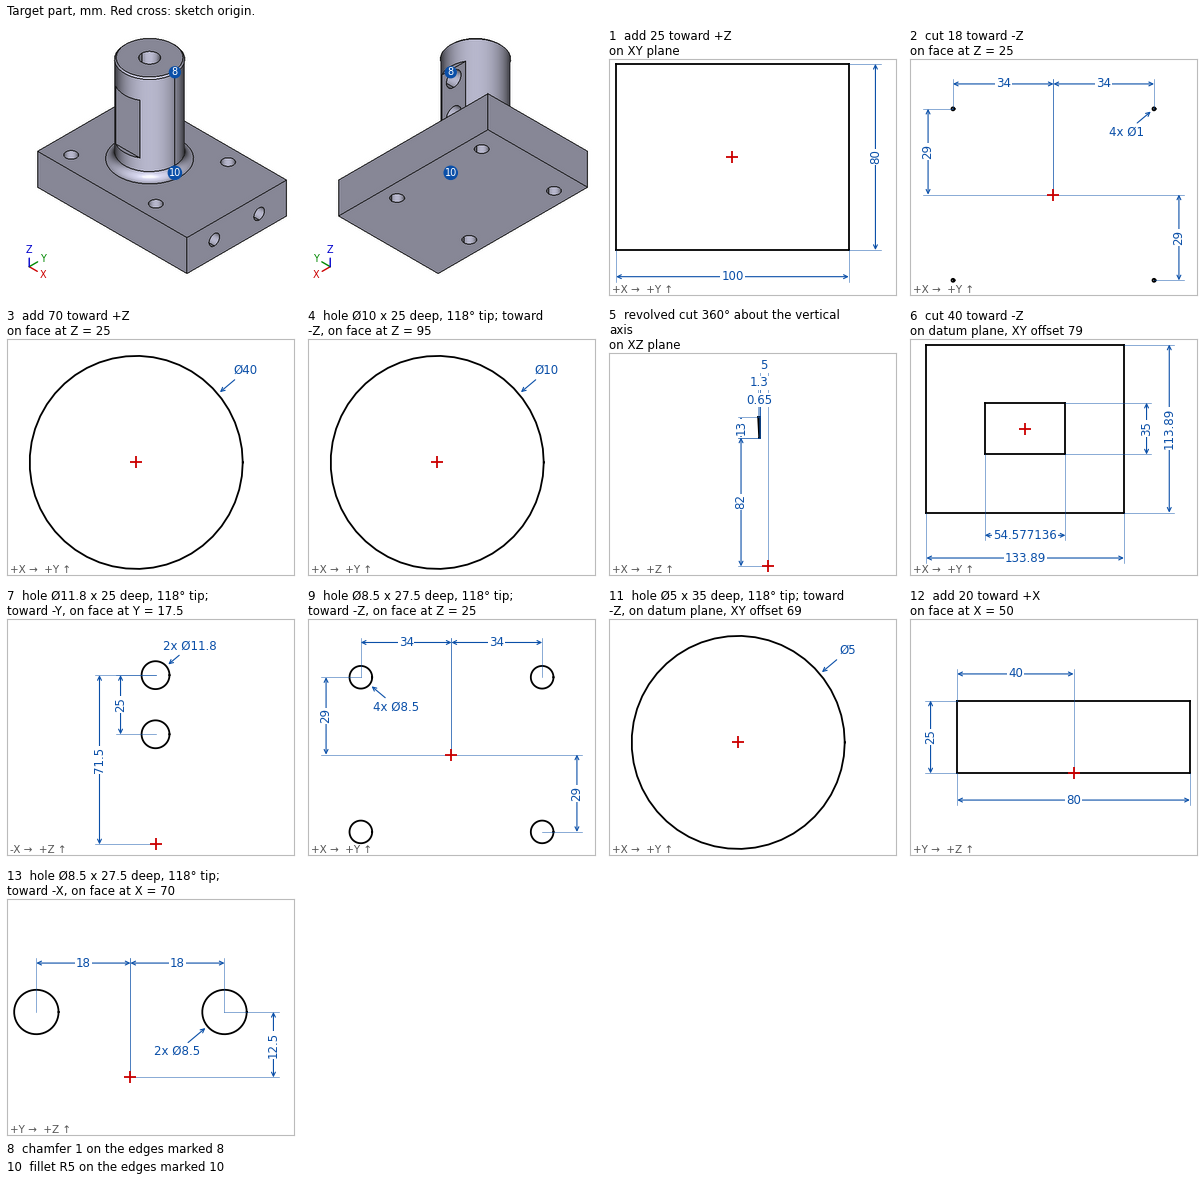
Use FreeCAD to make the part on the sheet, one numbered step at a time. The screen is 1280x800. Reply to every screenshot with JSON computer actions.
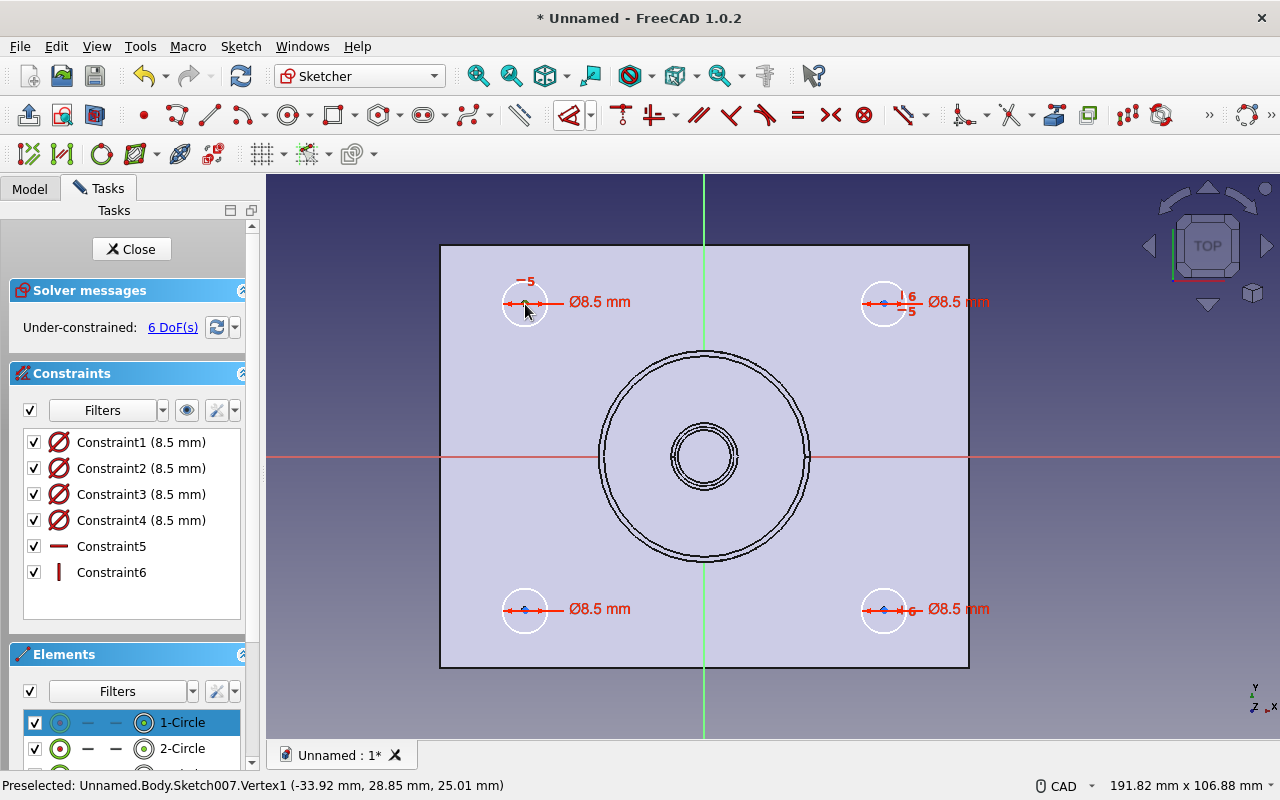
{"action": "left_click", "coordinate": [525, 611]}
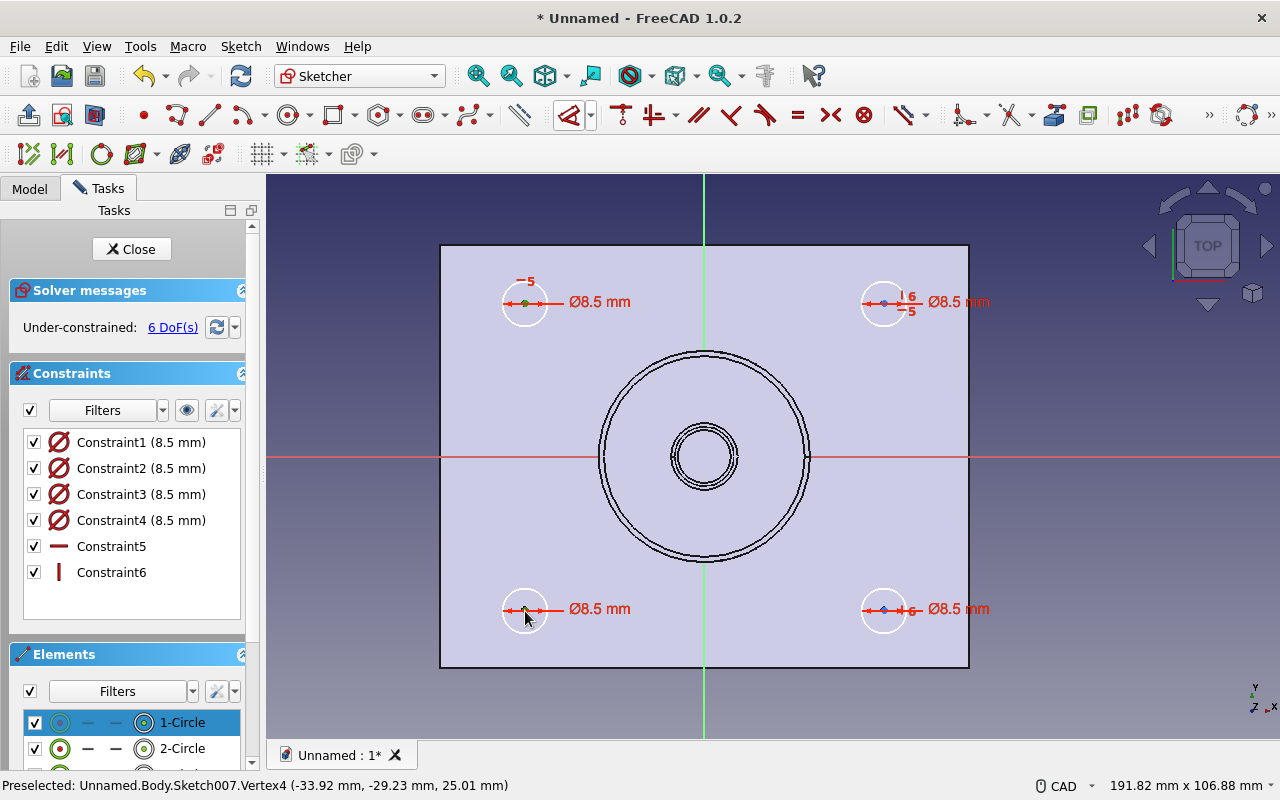
{"action": "key", "text": "v"}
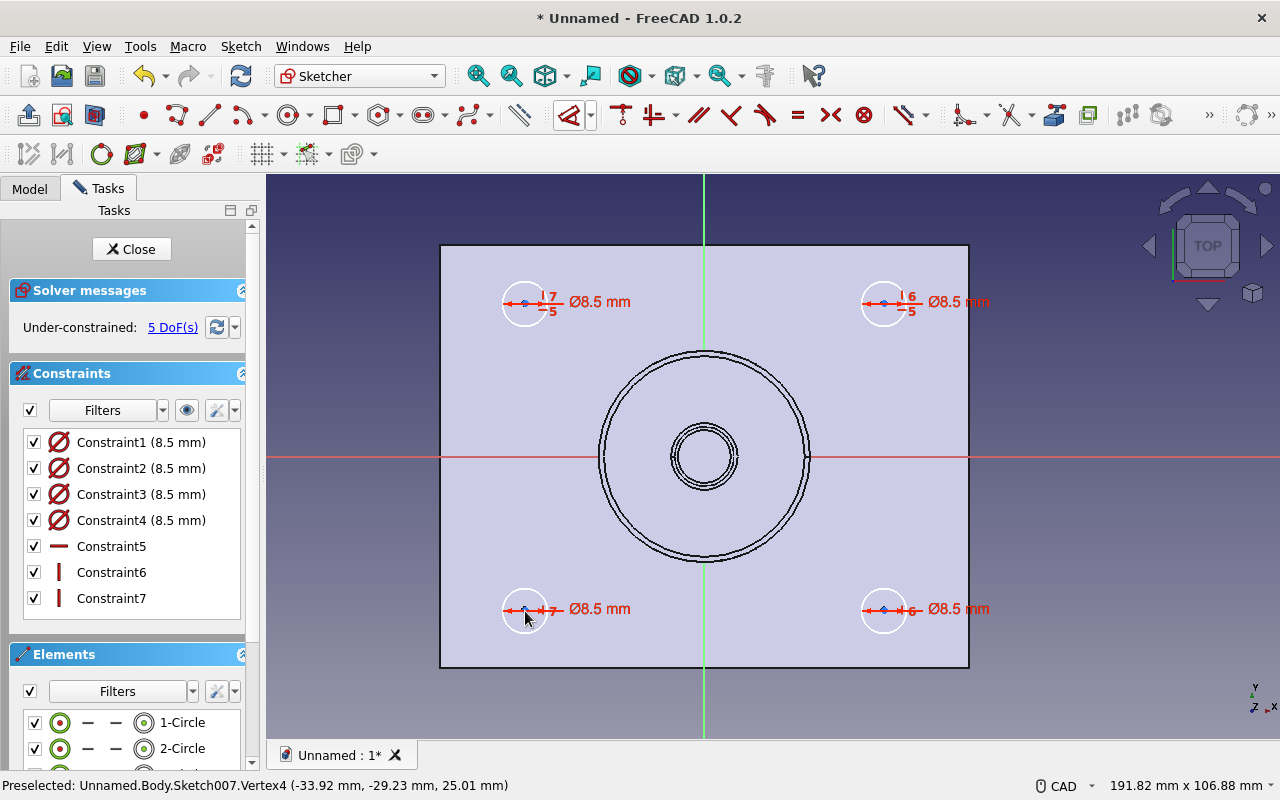
{"action": "left_click", "coordinate": [884, 611]}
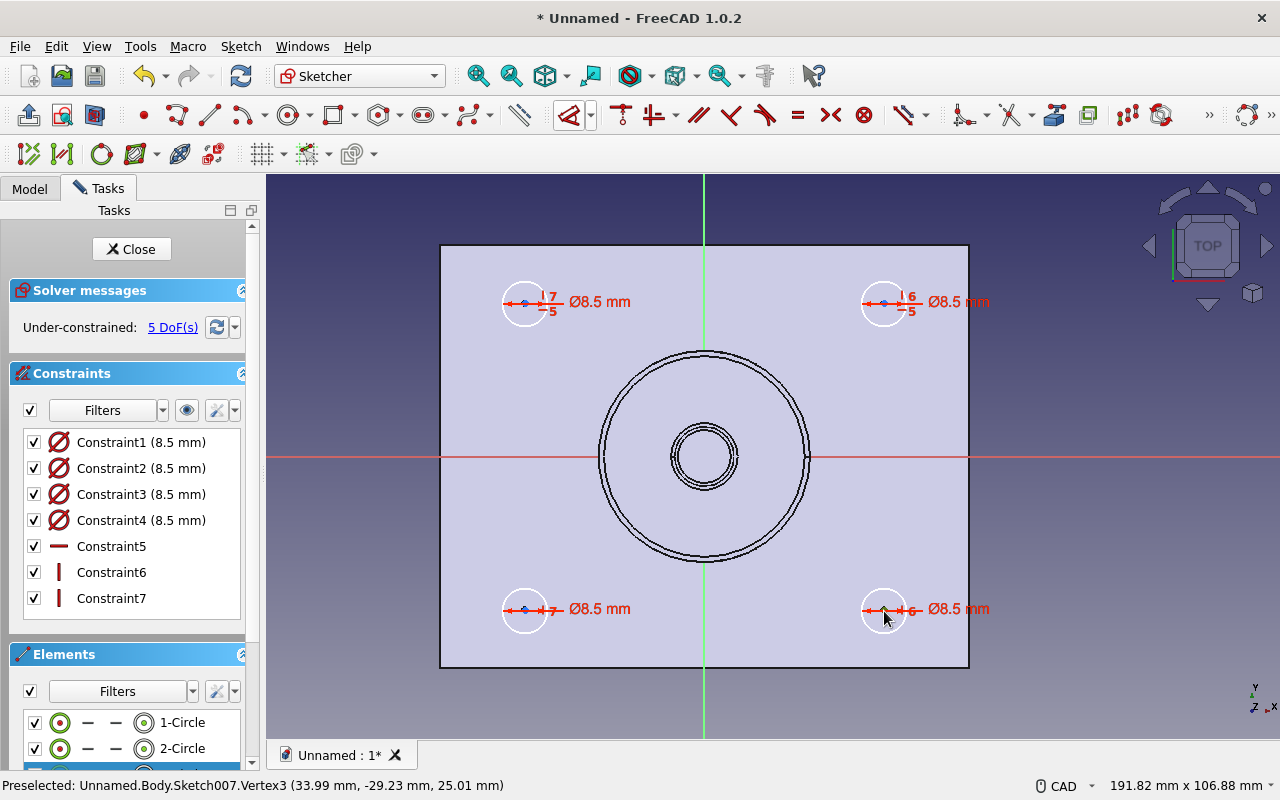
{"action": "left_click", "coordinate": [525, 611]}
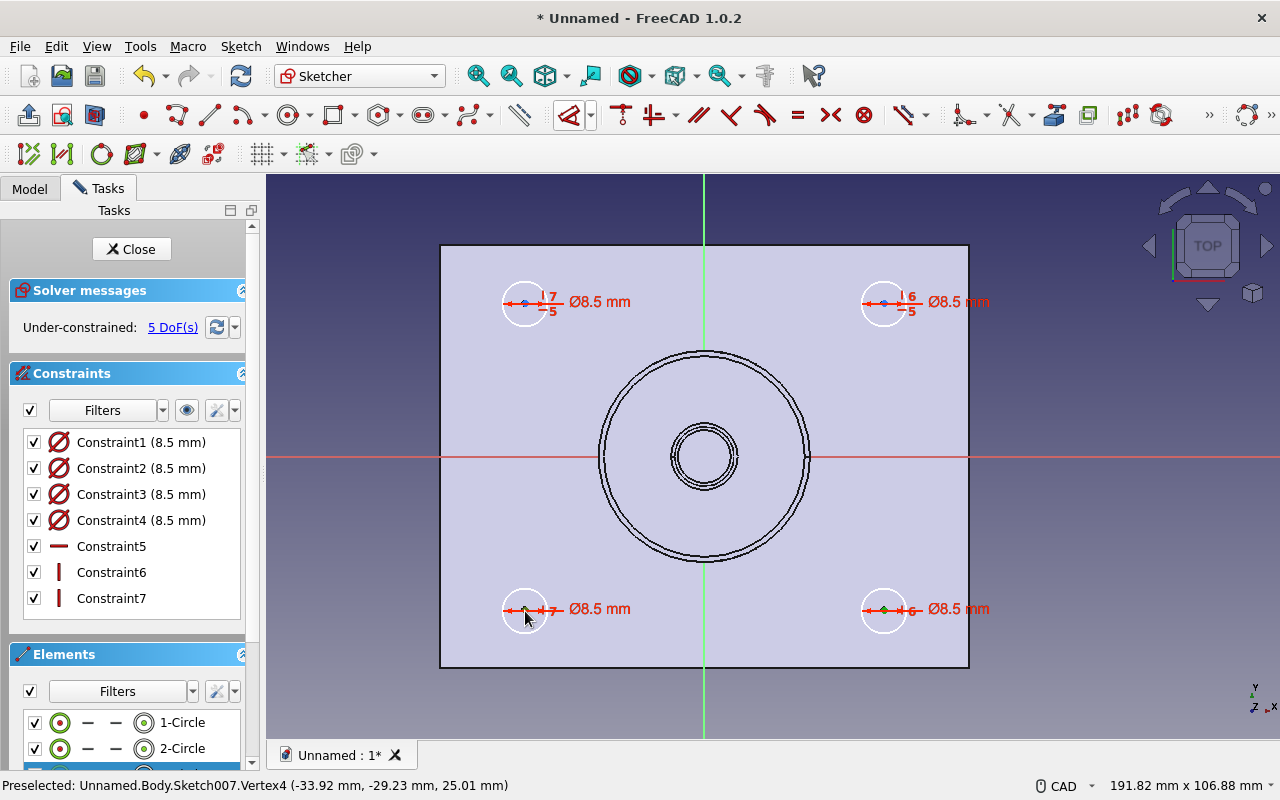
{"action": "left_click", "coordinate": [676, 116]}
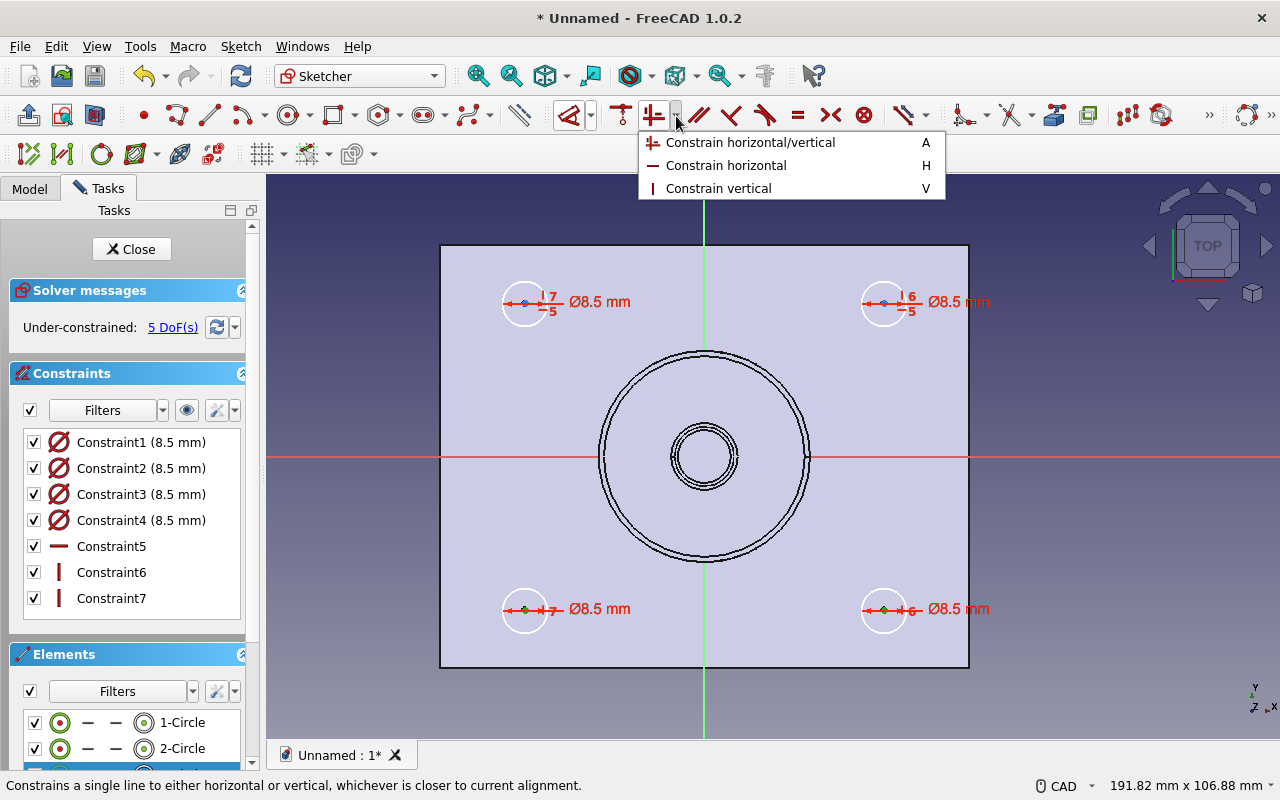
{"action": "left_click", "coordinate": [792, 166]}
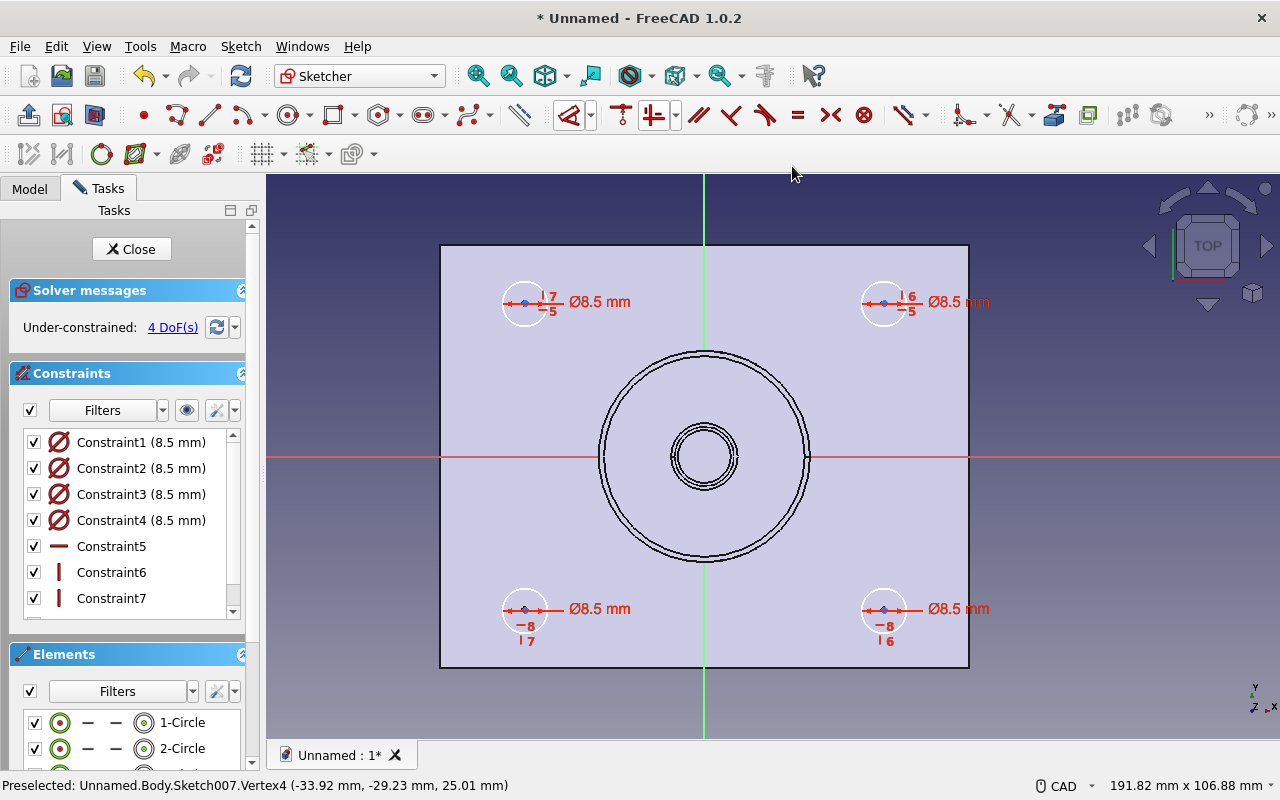
{"action": "left_click", "coordinate": [525, 304]}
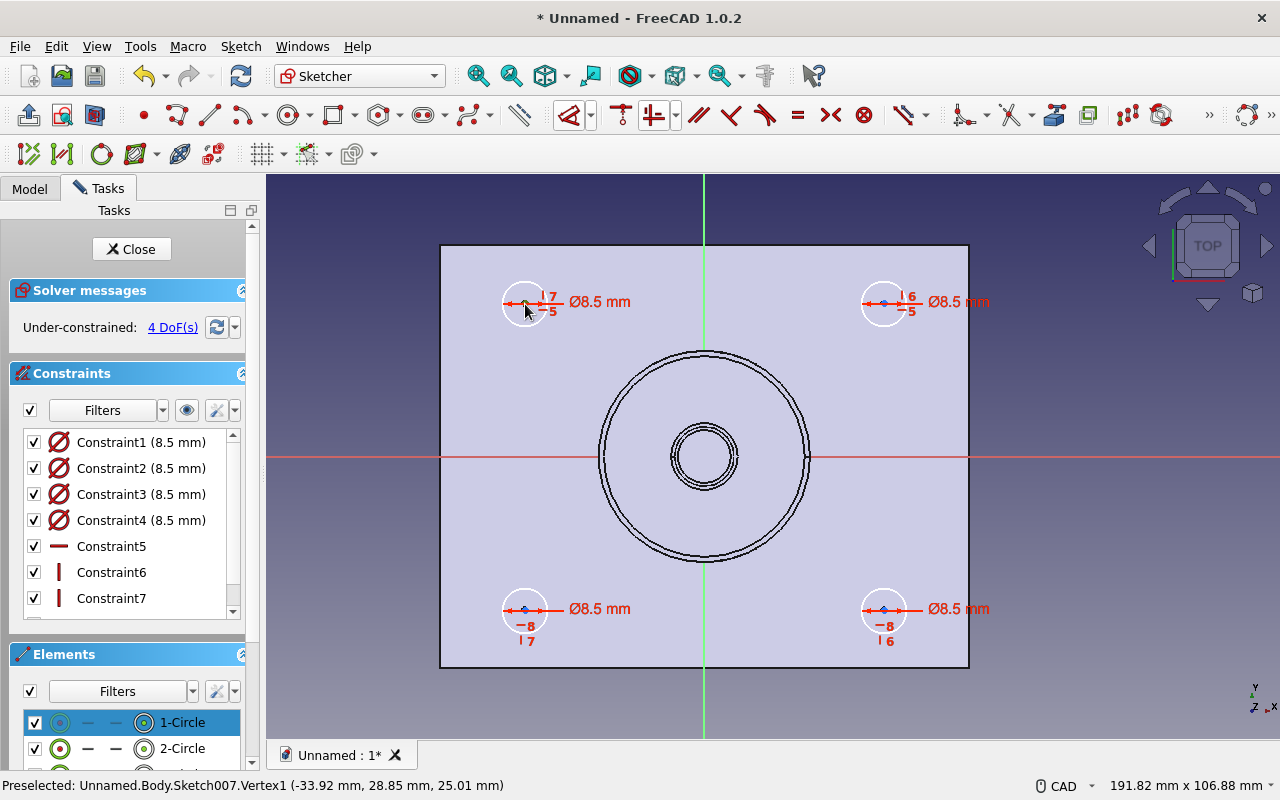
{"action": "key", "text": "l"}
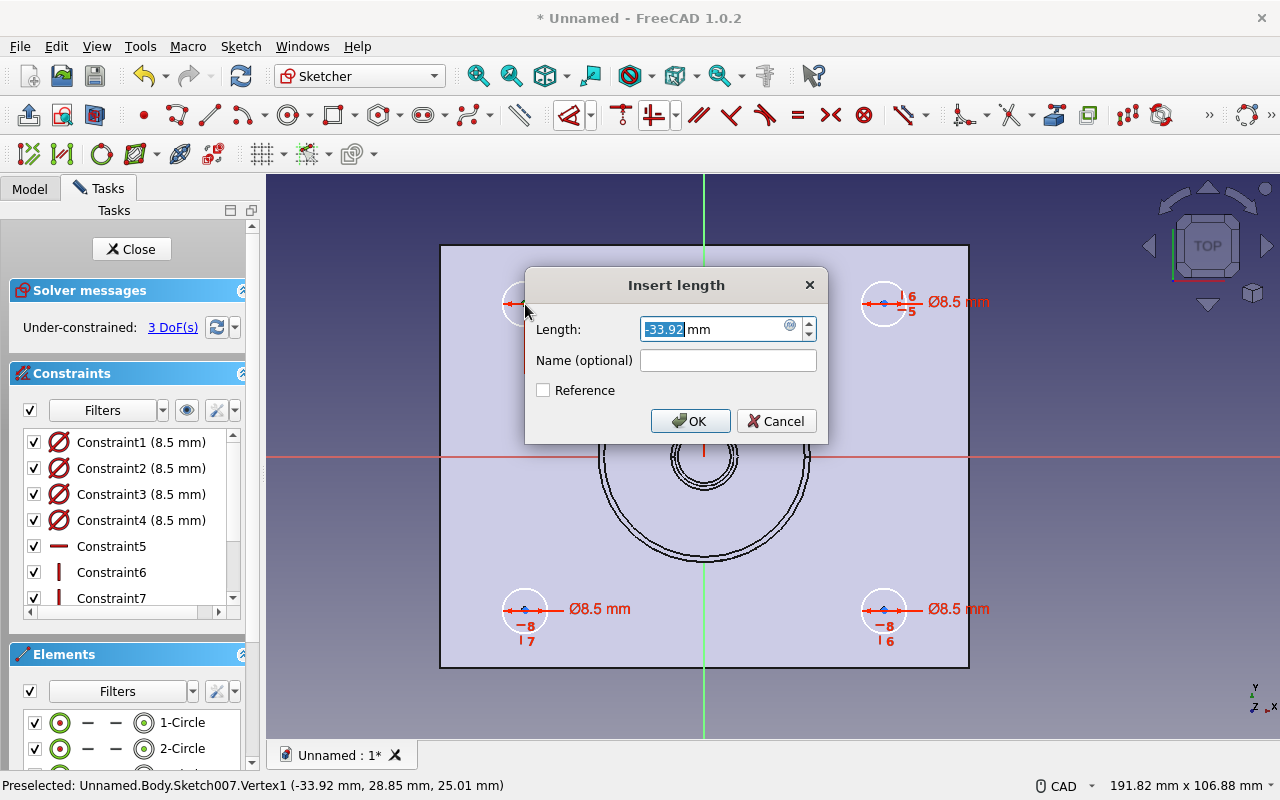
{"action": "type", "text": "-34"}
{"action": "key", "text": "Return"}